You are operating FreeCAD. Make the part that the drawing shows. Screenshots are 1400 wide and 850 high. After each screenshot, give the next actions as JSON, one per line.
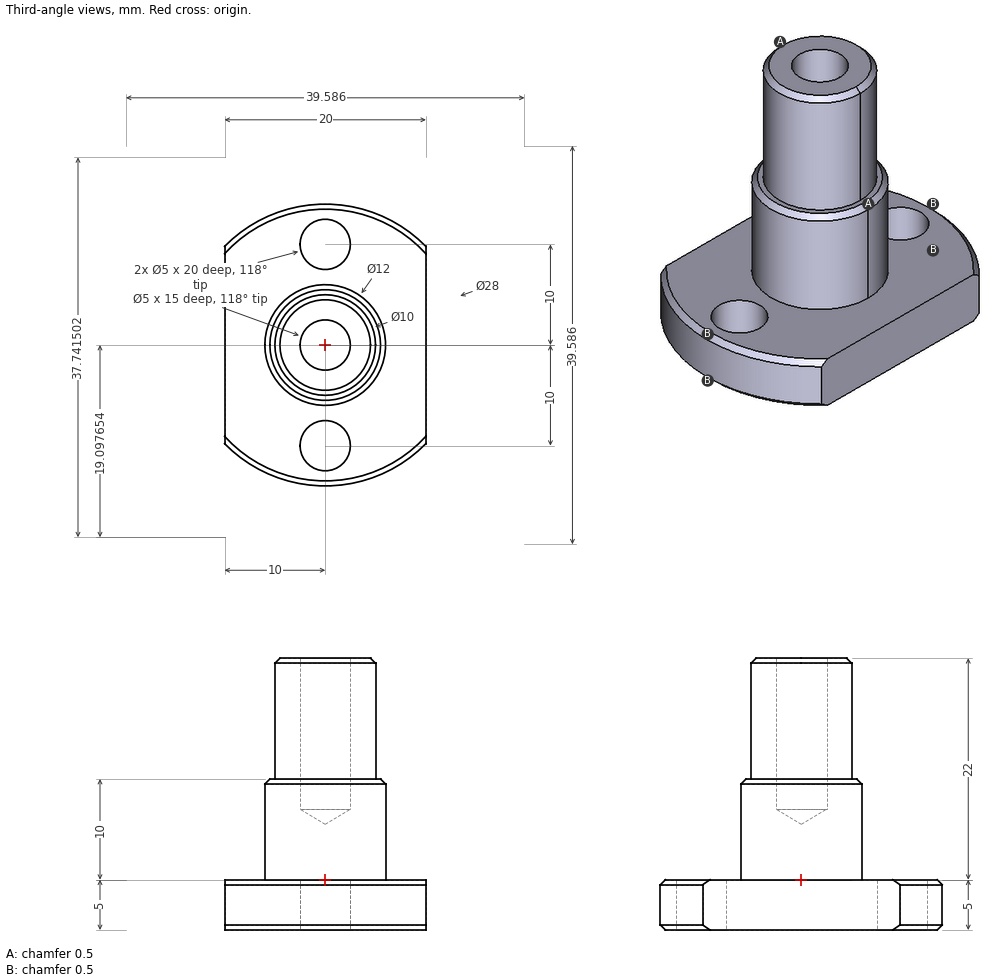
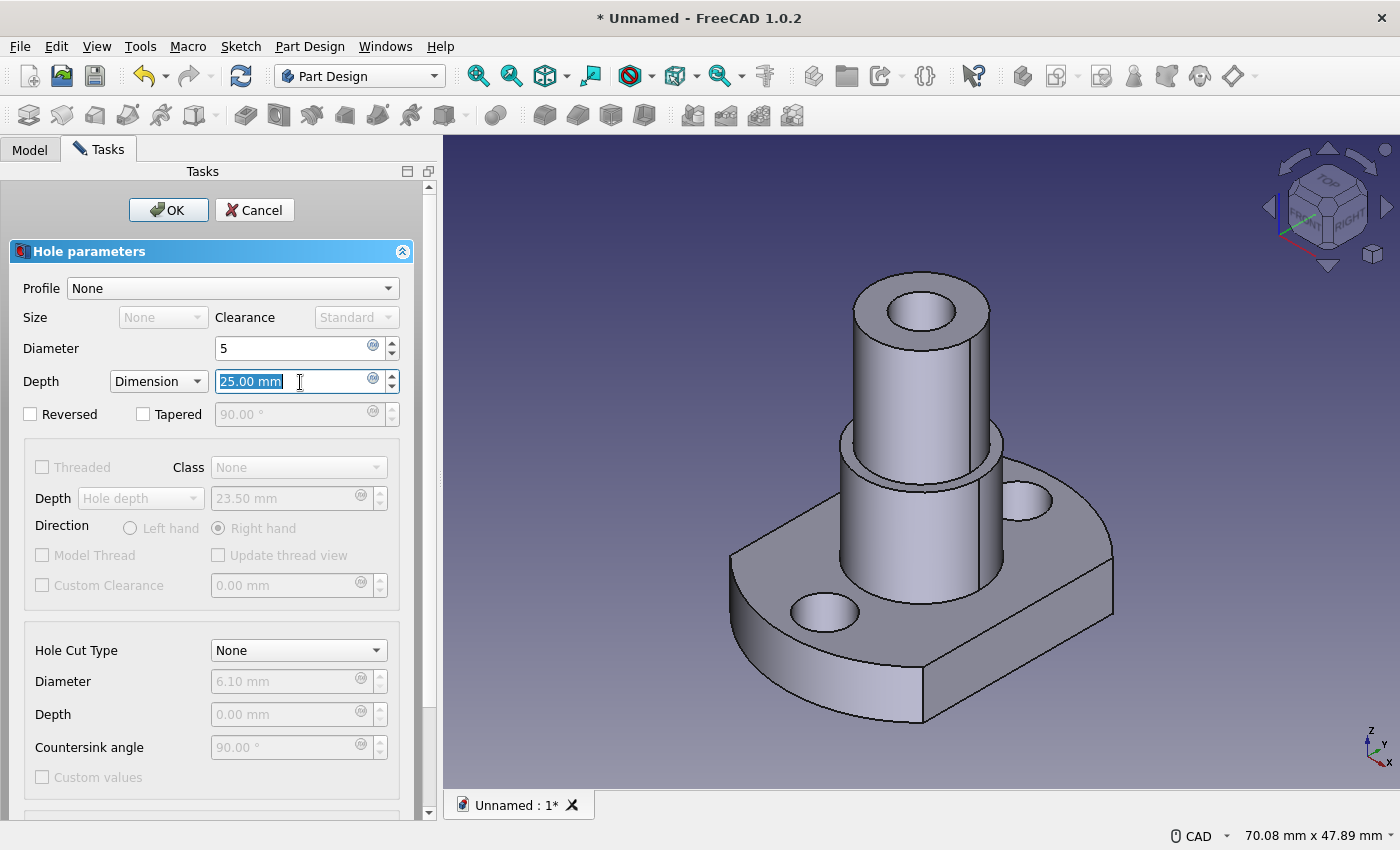
{"action": "type", "text": "15"}
{"action": "key", "text": "Tab"}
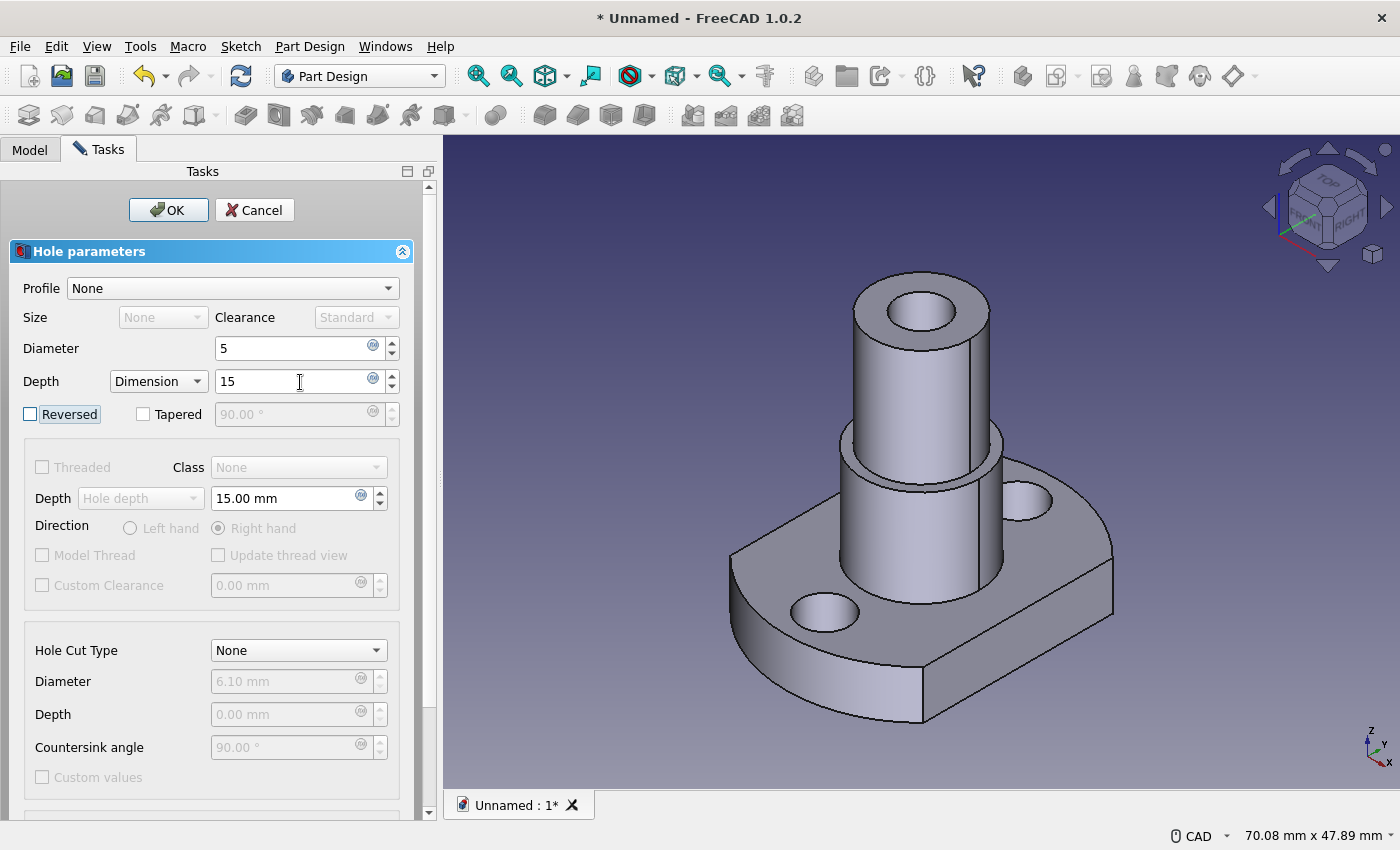
{"action": "left_click", "coordinate": [169, 210]}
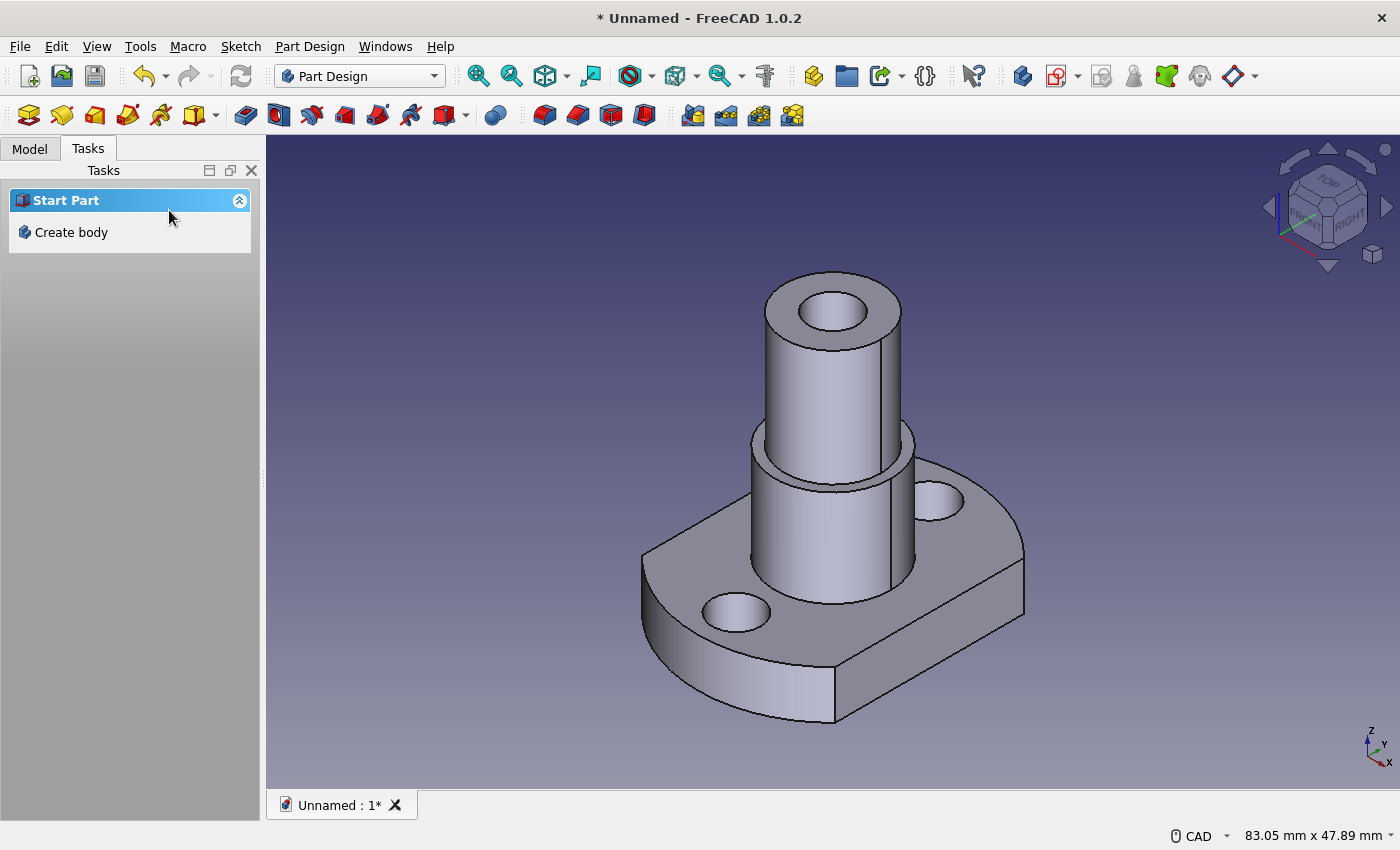
{"action": "left_click", "coordinate": [772, 328]}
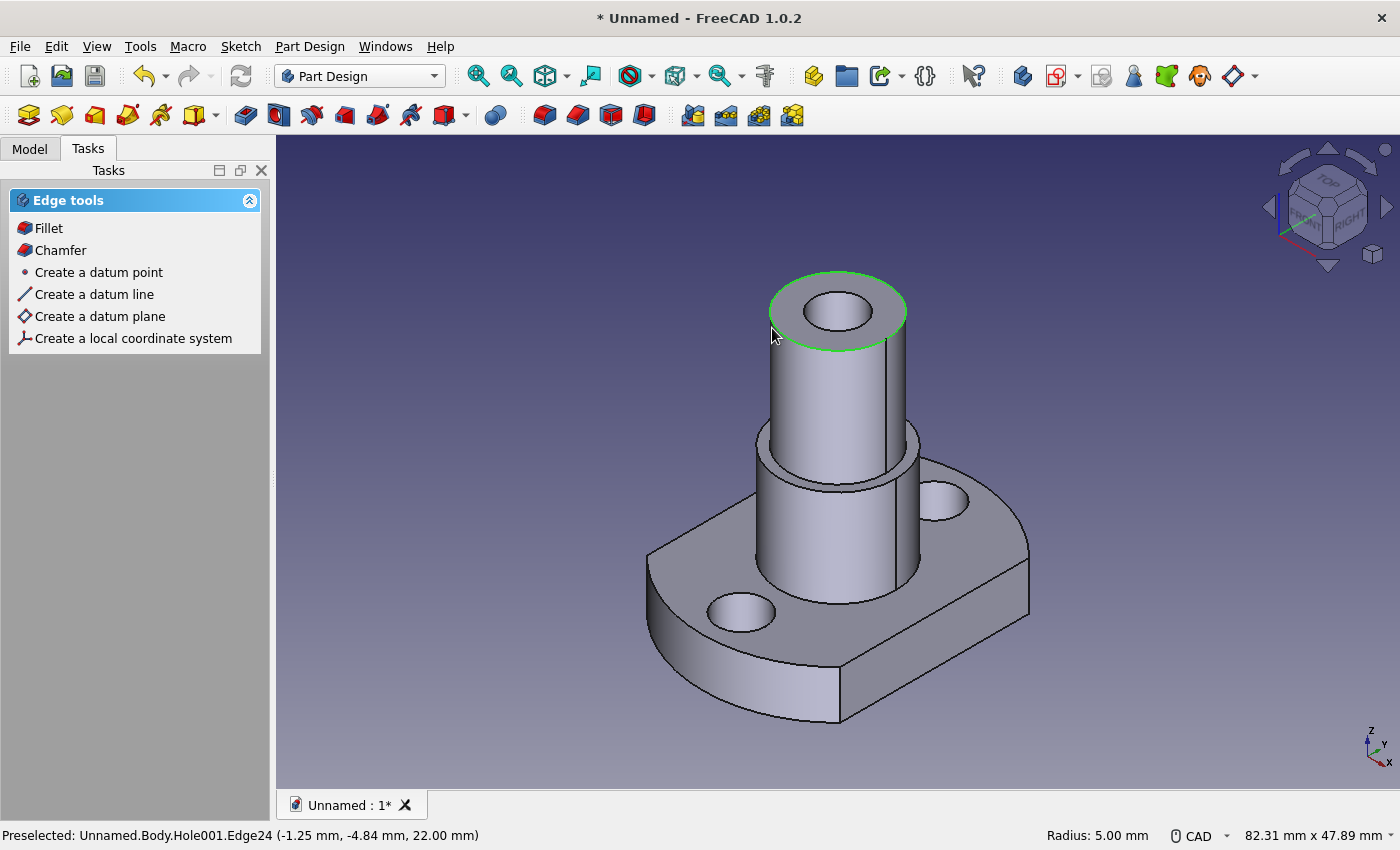
{"action": "left_click", "coordinate": [765, 466], "text": "ctrl"}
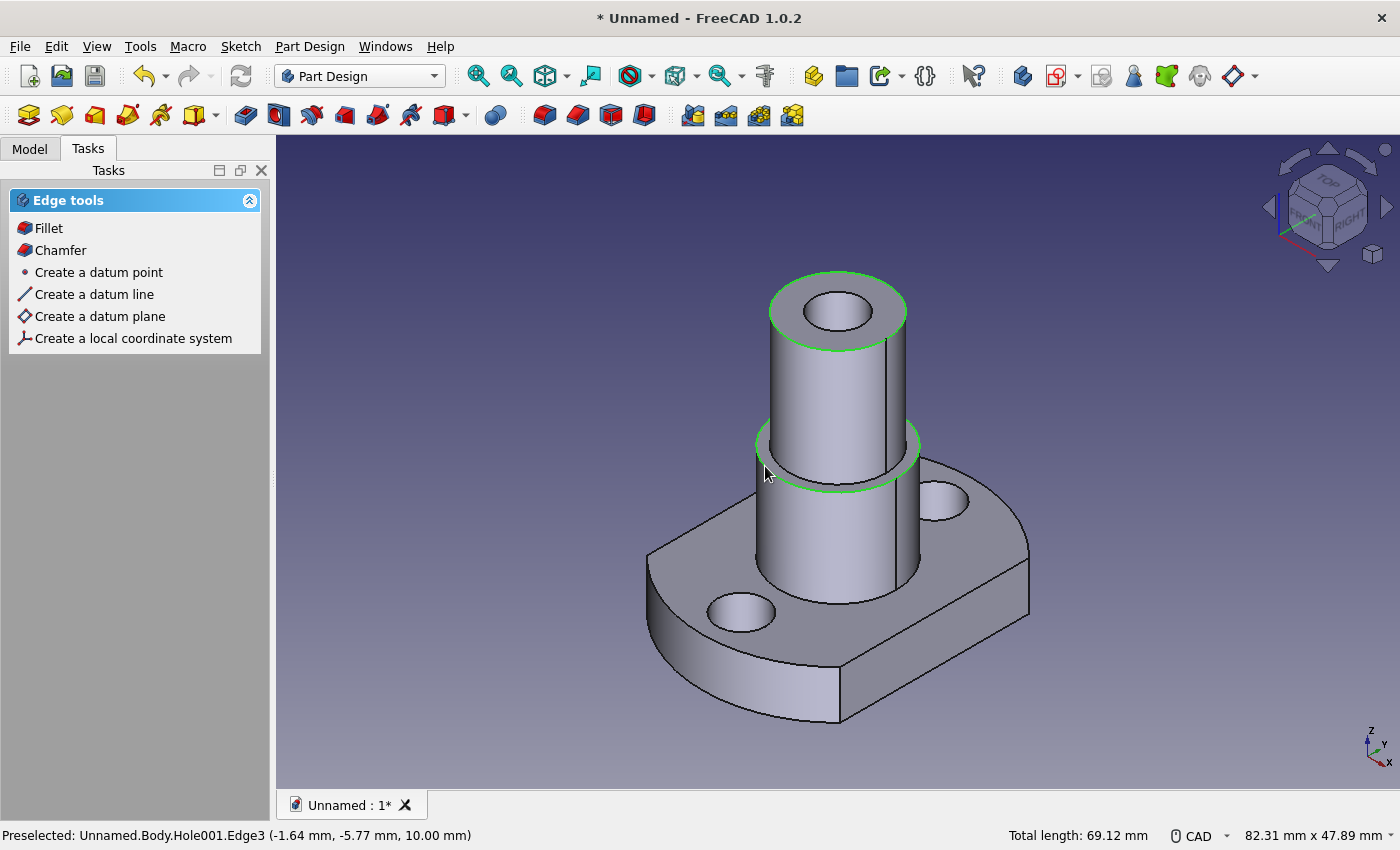
{"action": "left_click", "coordinate": [578, 116]}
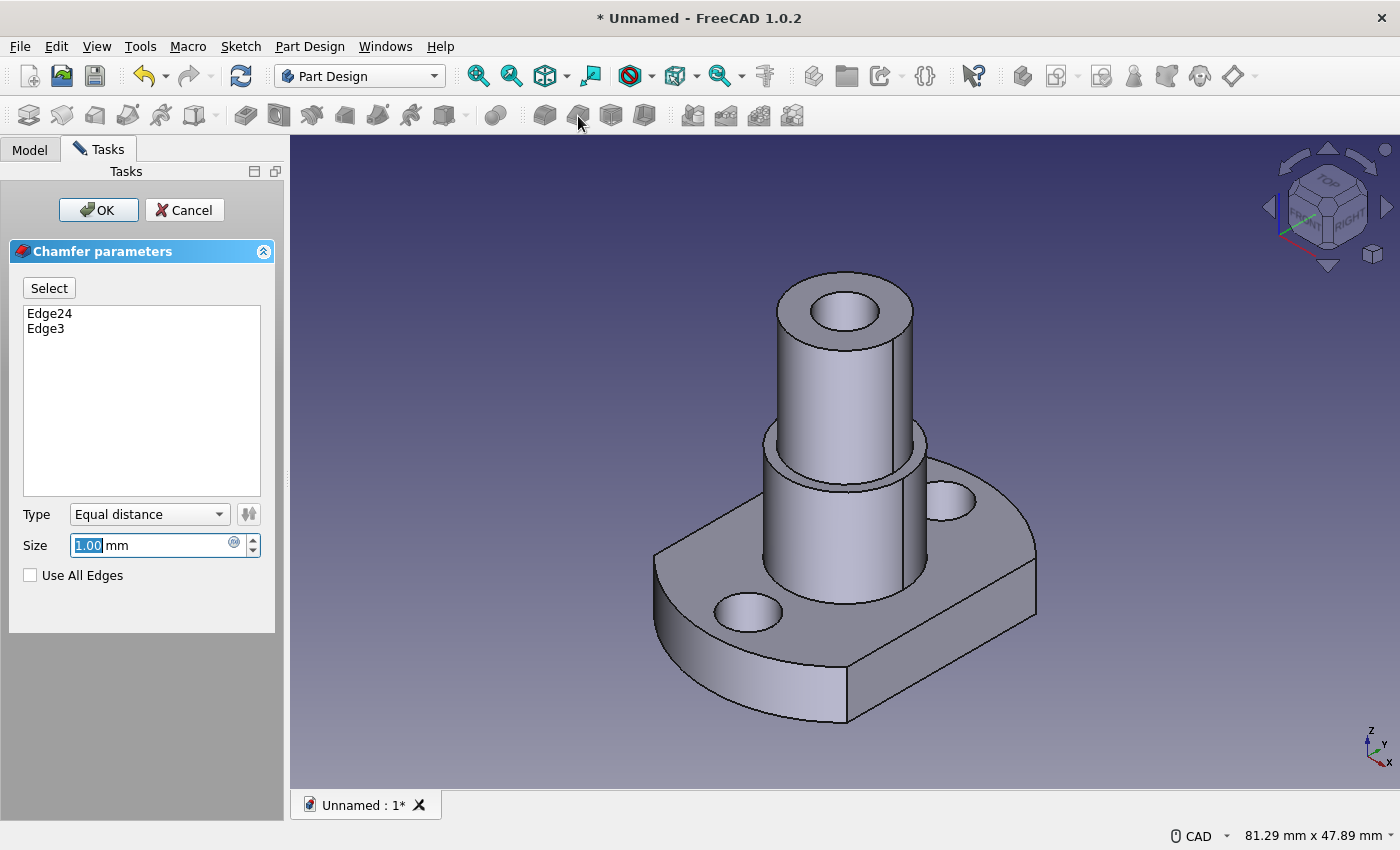
{"action": "type", "text": "0.5"}
{"action": "key", "text": "Tab"}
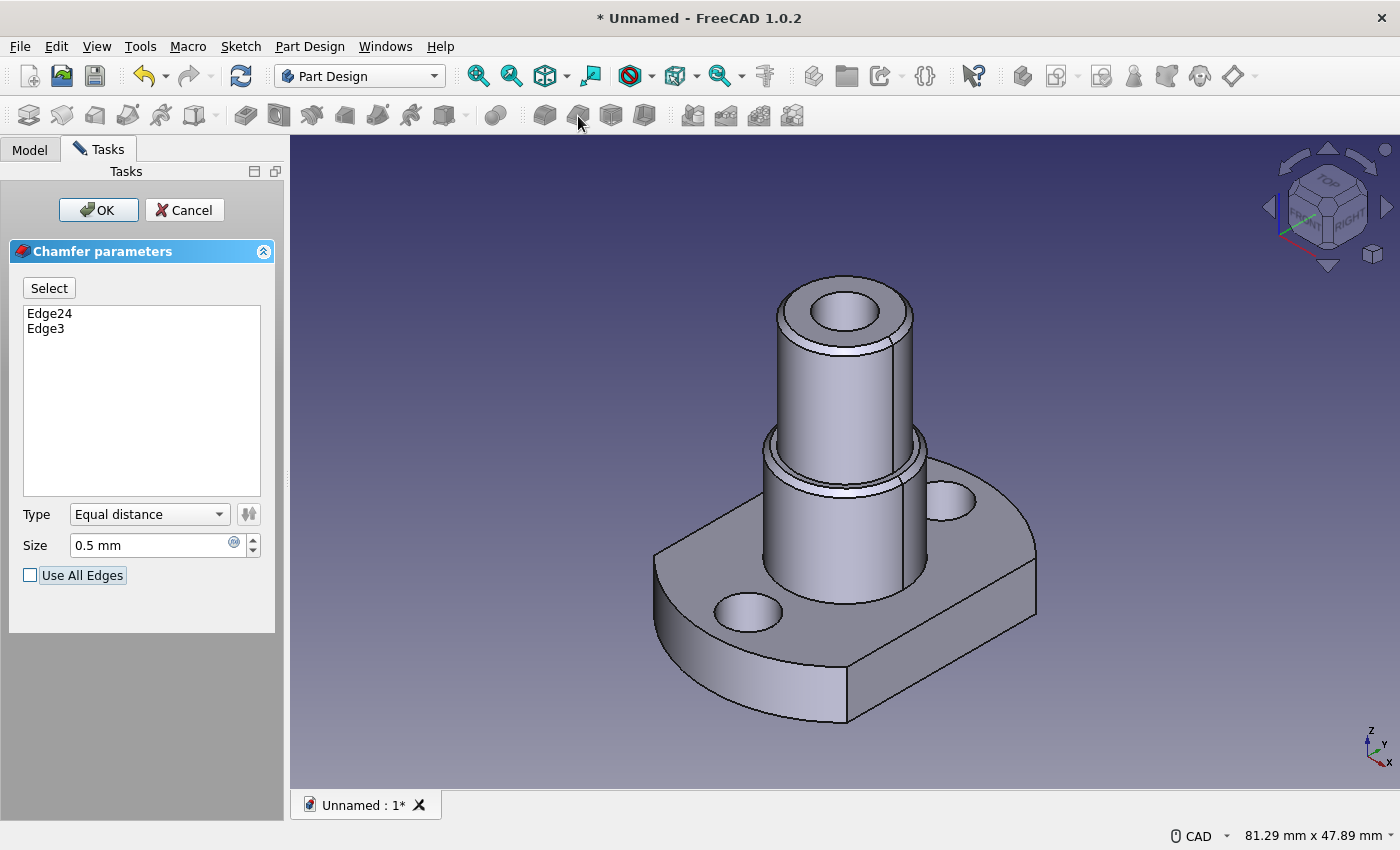
{"action": "left_click", "coordinate": [99, 210]}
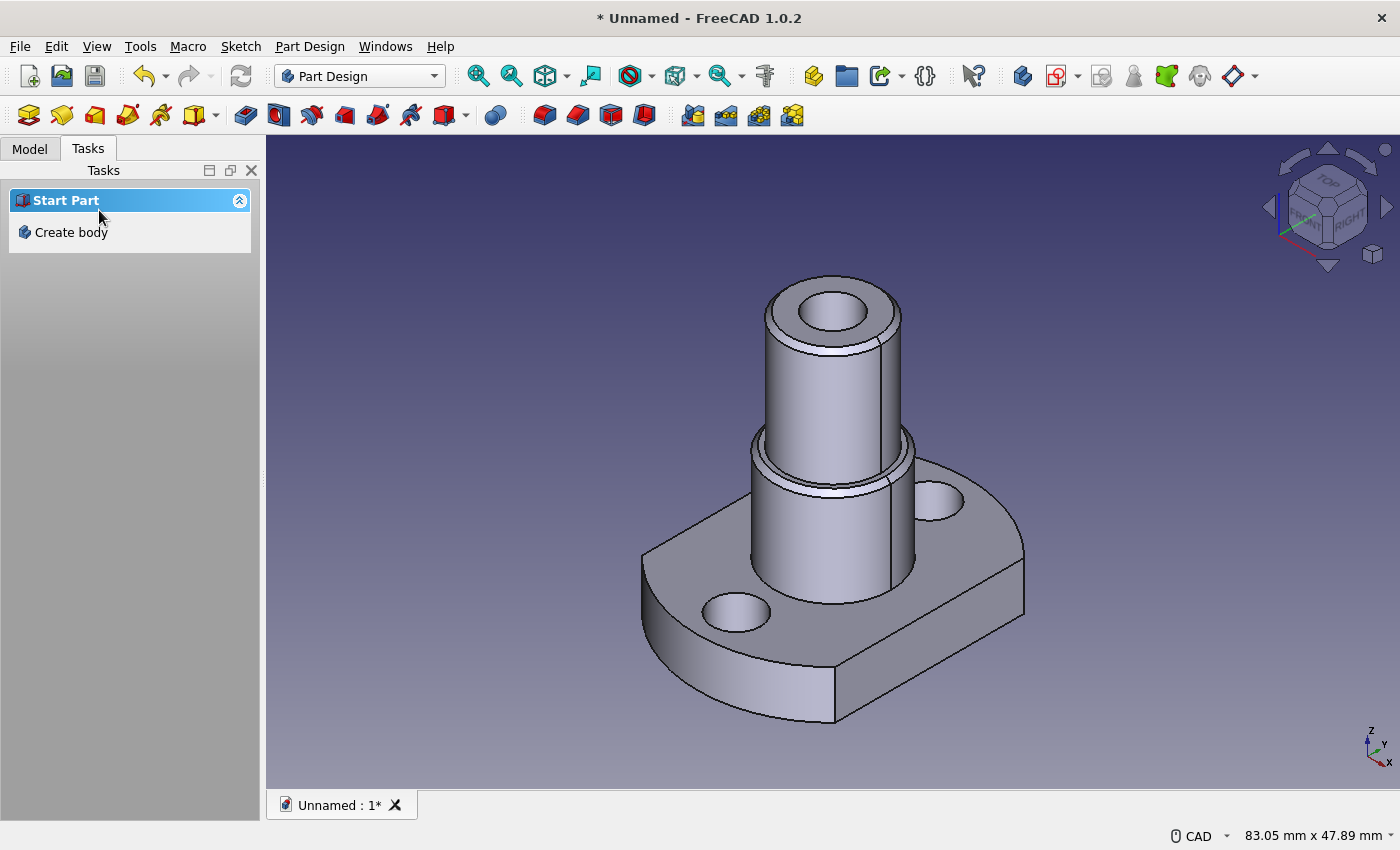
{"action": "left_click", "coordinate": [1004, 506]}